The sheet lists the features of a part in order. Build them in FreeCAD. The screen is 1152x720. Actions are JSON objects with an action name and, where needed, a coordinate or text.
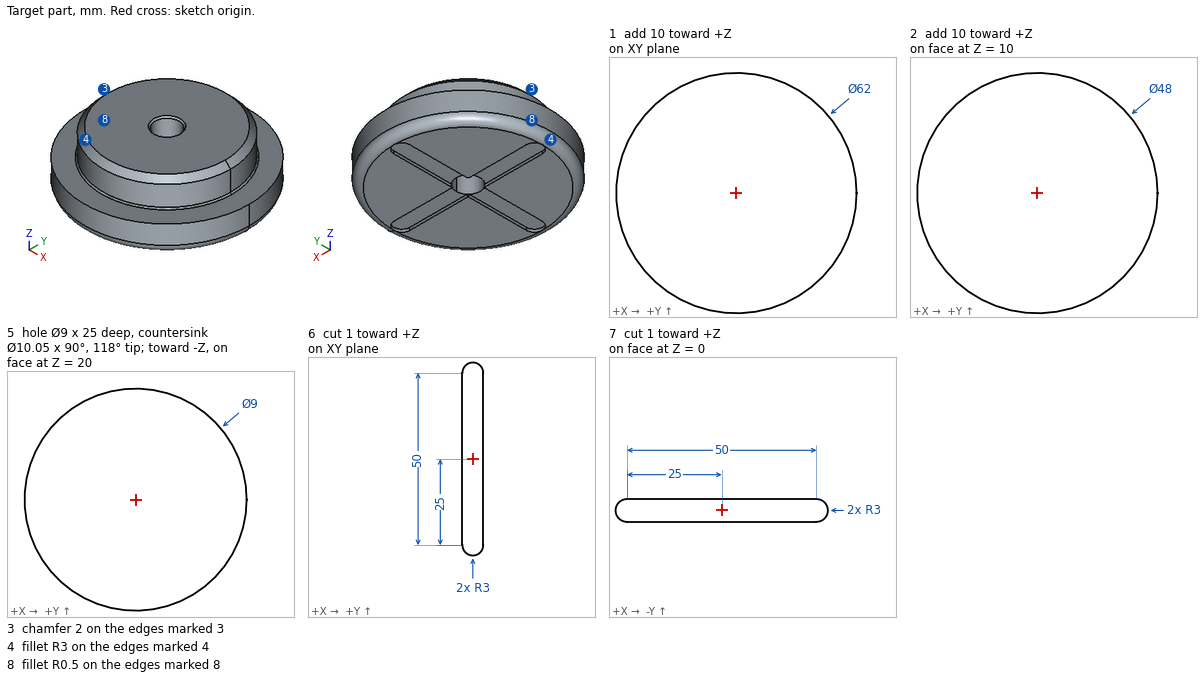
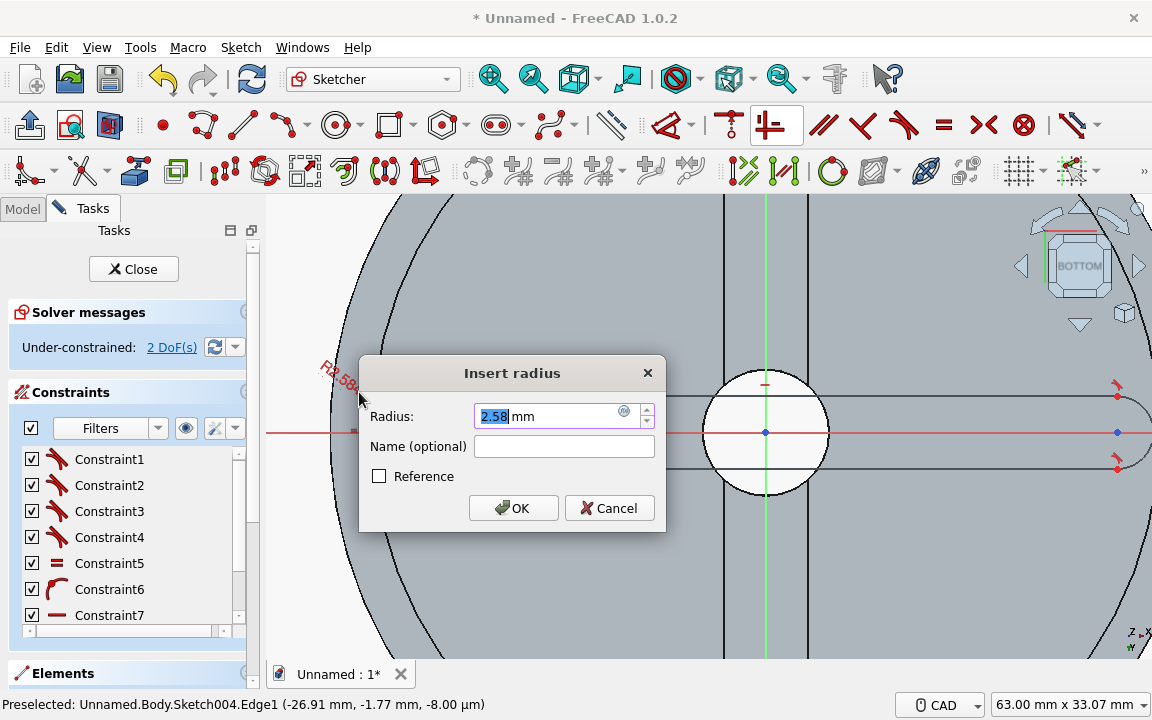
{"action": "type", "text": "3"}
{"action": "key", "text": "Return"}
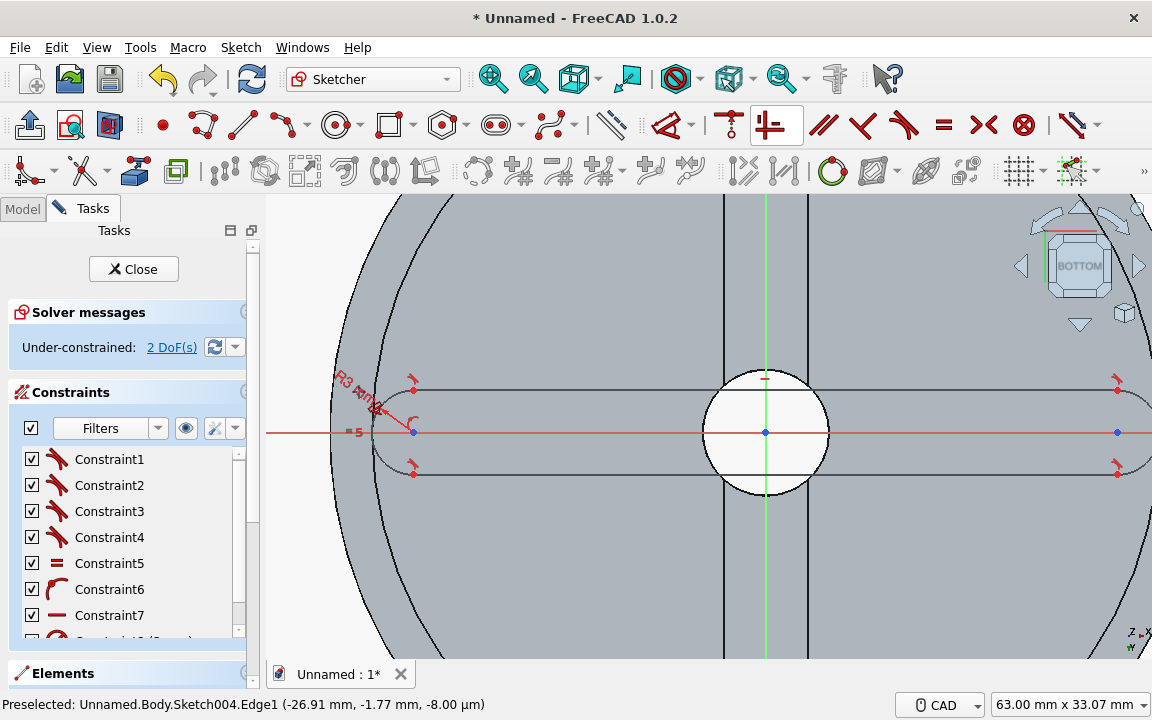
{"action": "left_click", "coordinate": [625, 390]}
{"action": "left_click", "coordinate": [700, 356]}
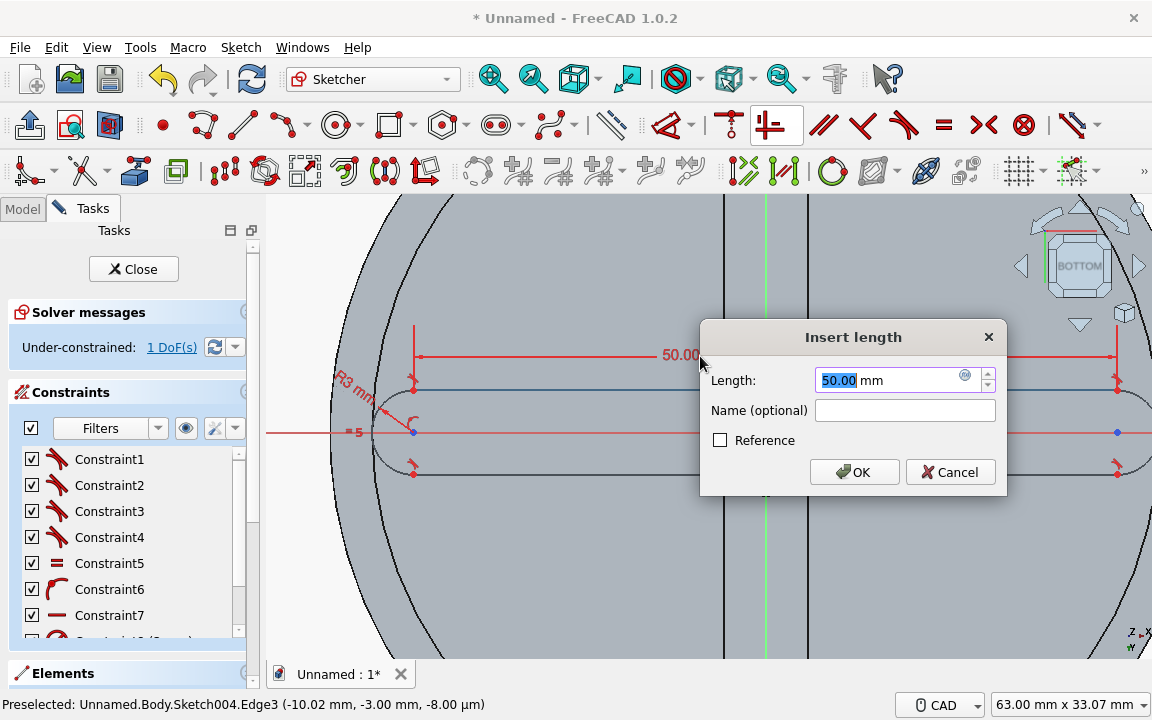
{"action": "type", "text": "50"}
{"action": "key", "text": "Return"}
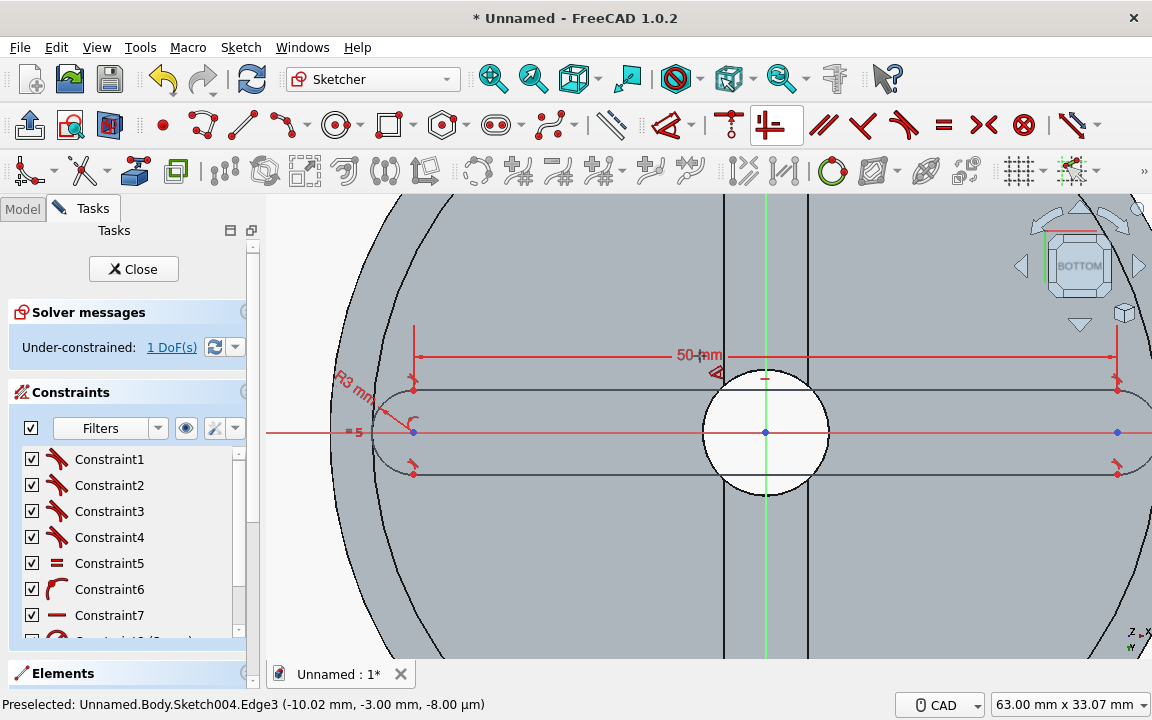
{"action": "left_click", "coordinate": [414, 390]}
{"action": "left_click", "coordinate": [590, 356]}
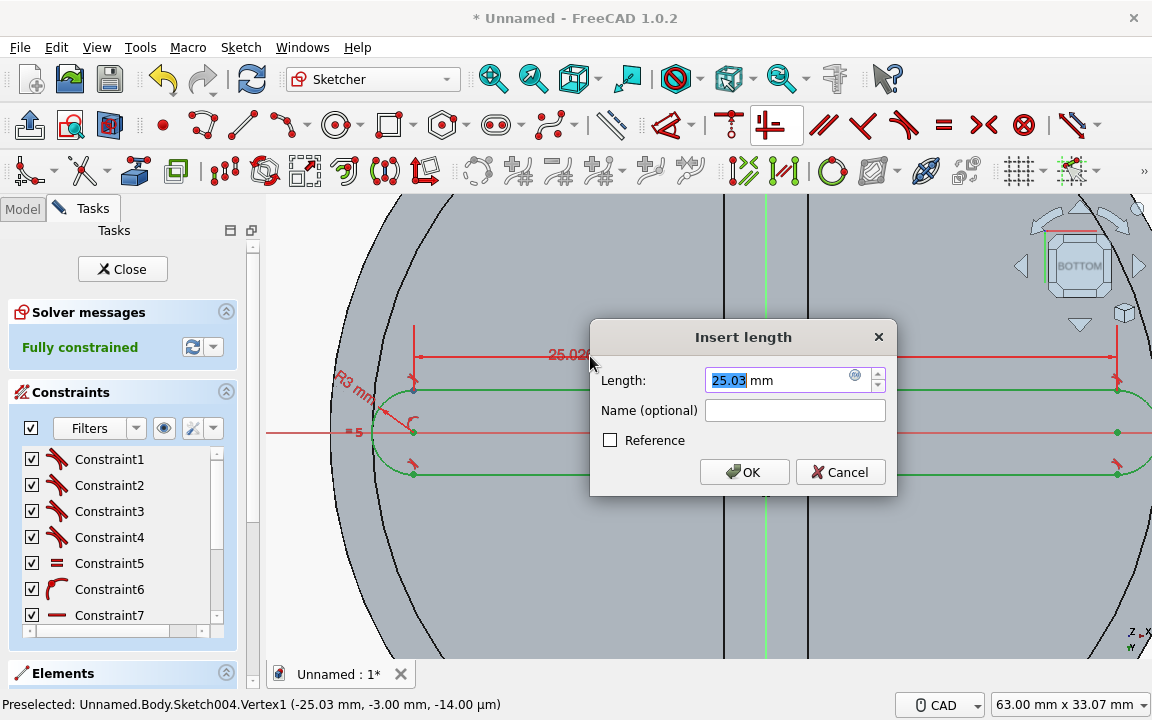
{"action": "type", "text": "25"}
{"action": "key", "text": "Return"}
{"action": "key", "text": "Escape"}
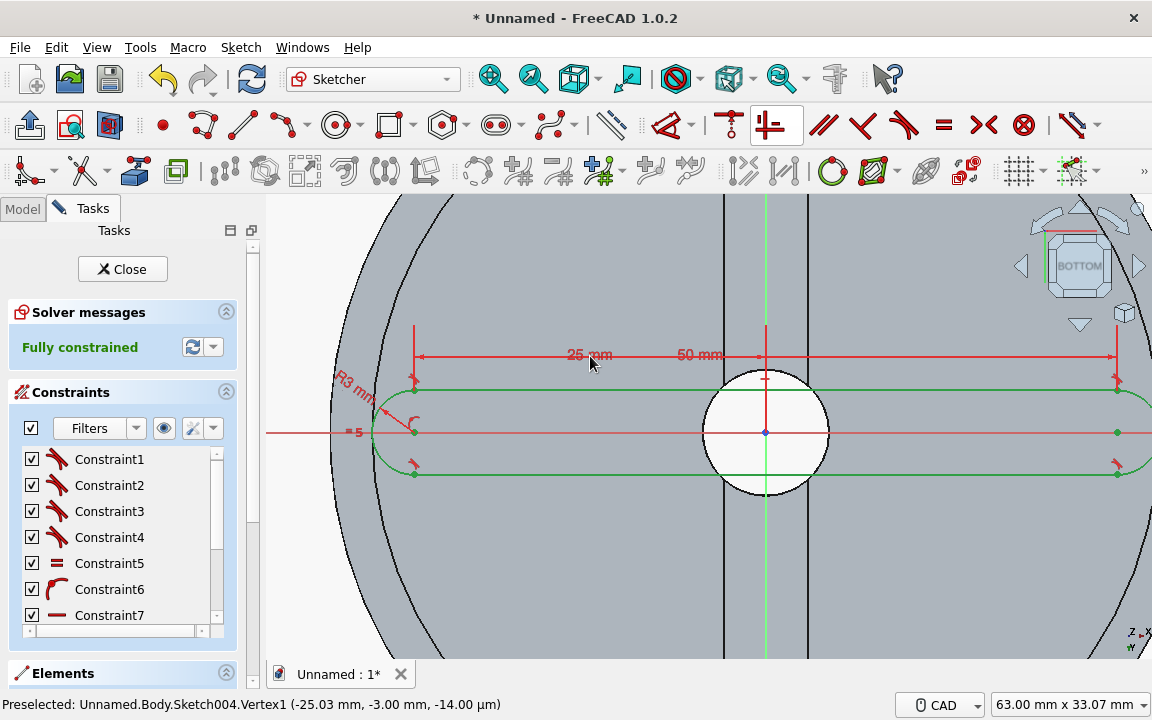
{"action": "left_click", "coordinate": [123, 269]}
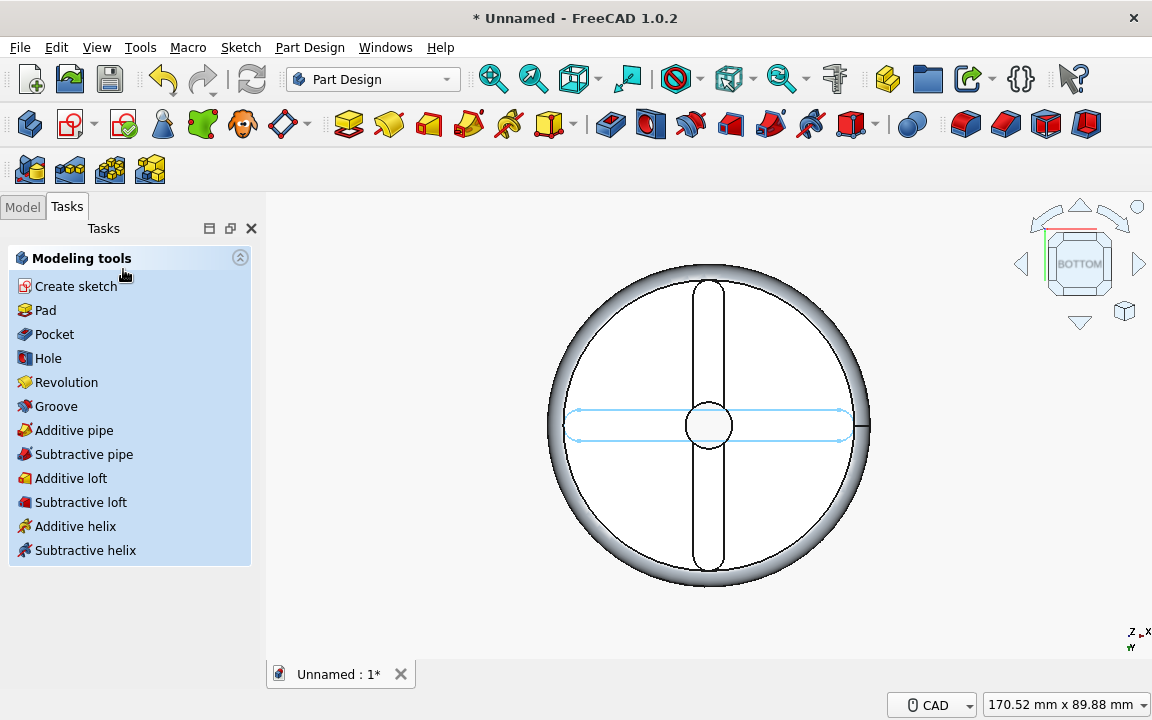
{"action": "left_click", "coordinate": [612, 124]}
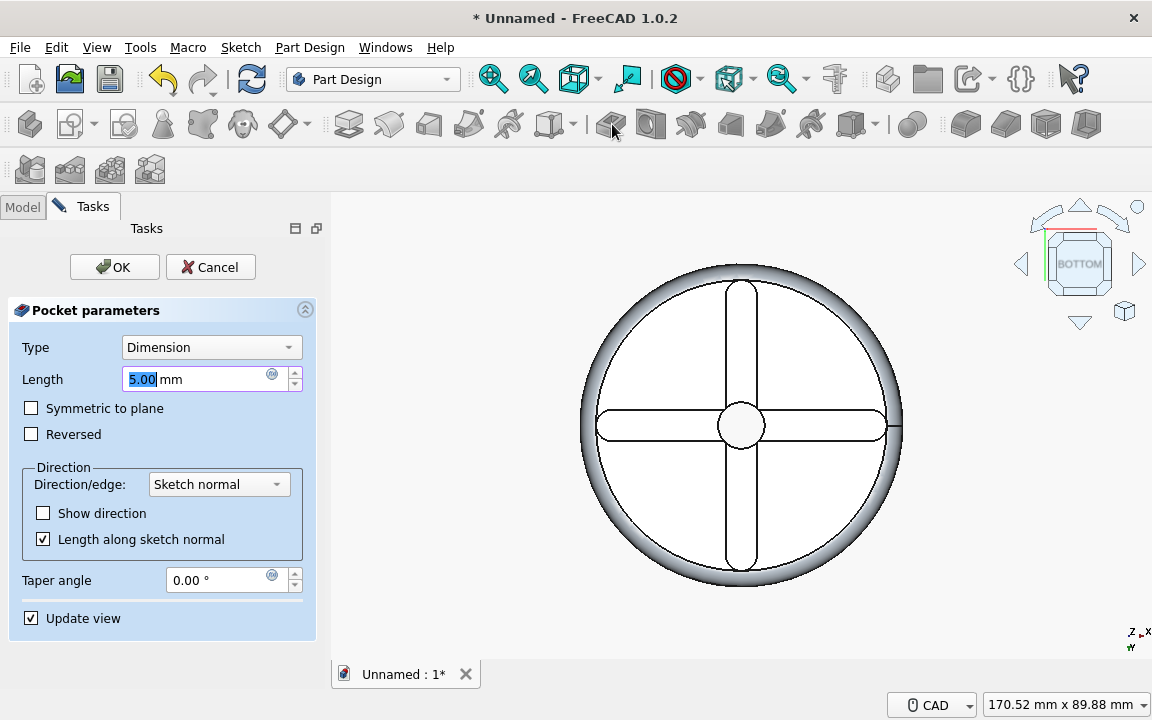
{"action": "type", "text": "1"}
{"action": "key", "text": "Tab"}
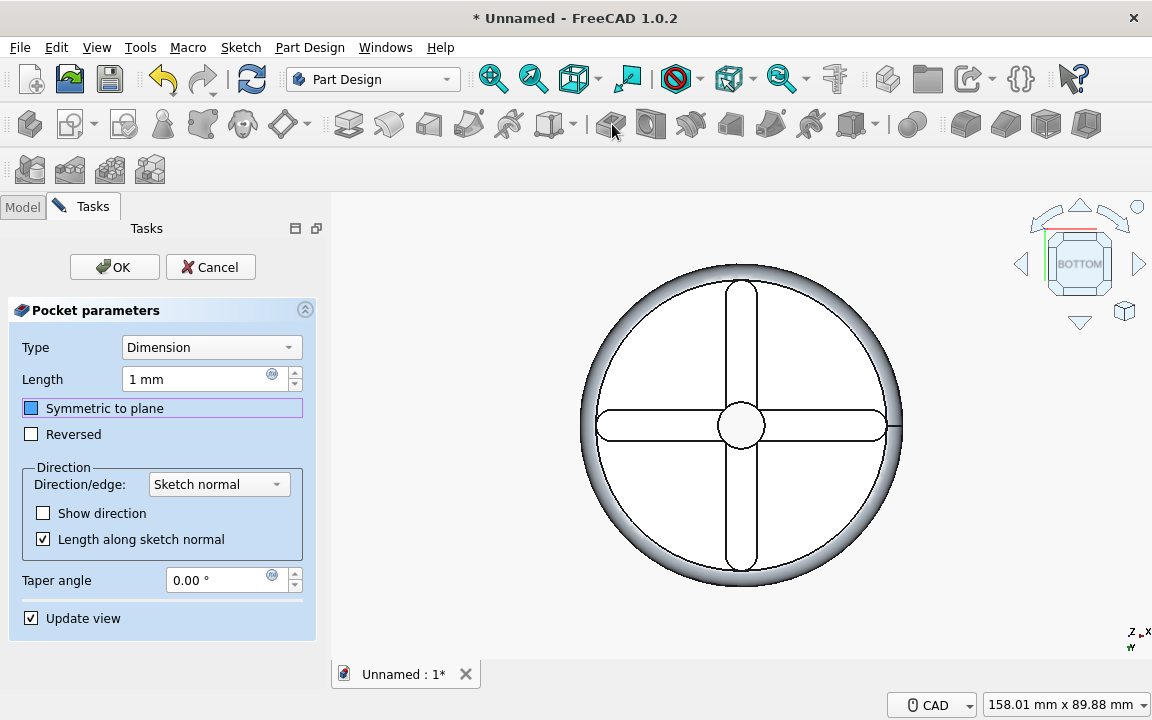
{"action": "left_click", "coordinate": [115, 267]}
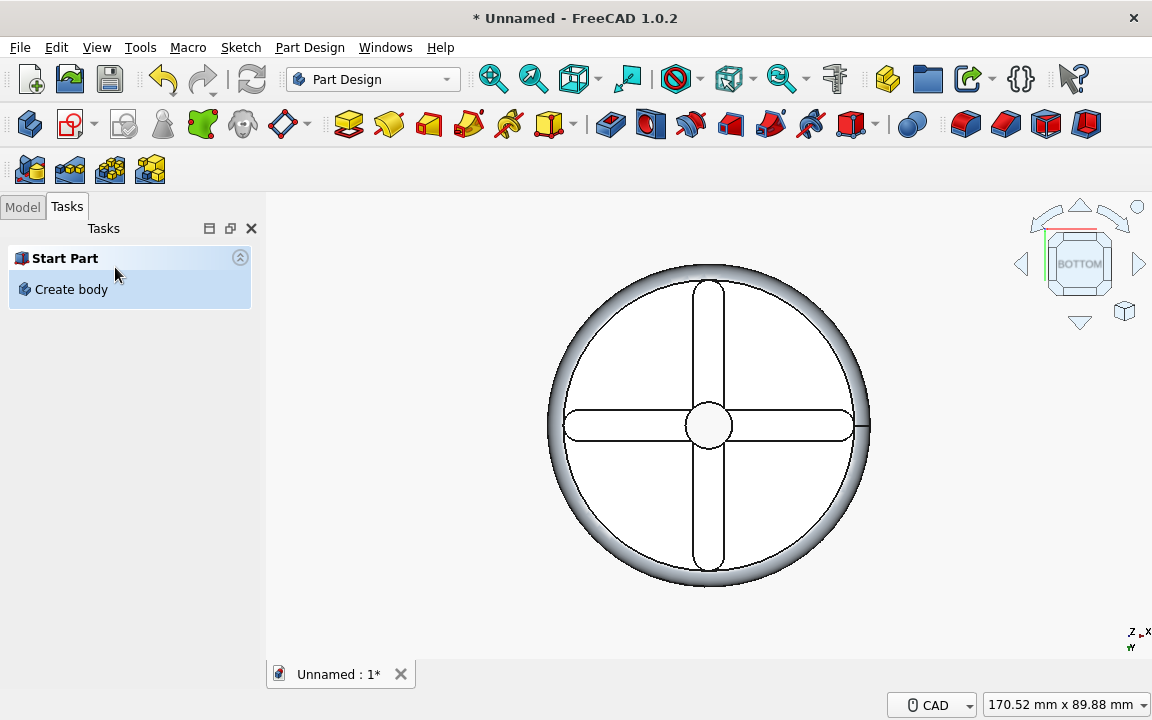
{"action": "key", "text": "0"}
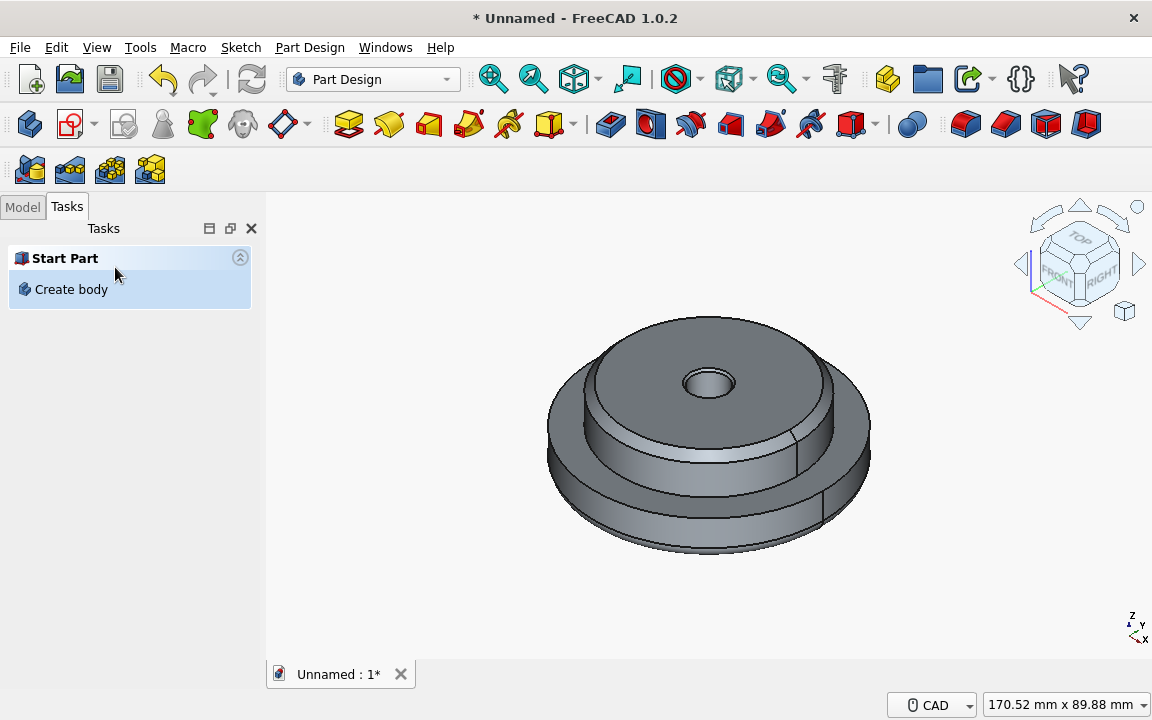
{"action": "key", "text": "2"}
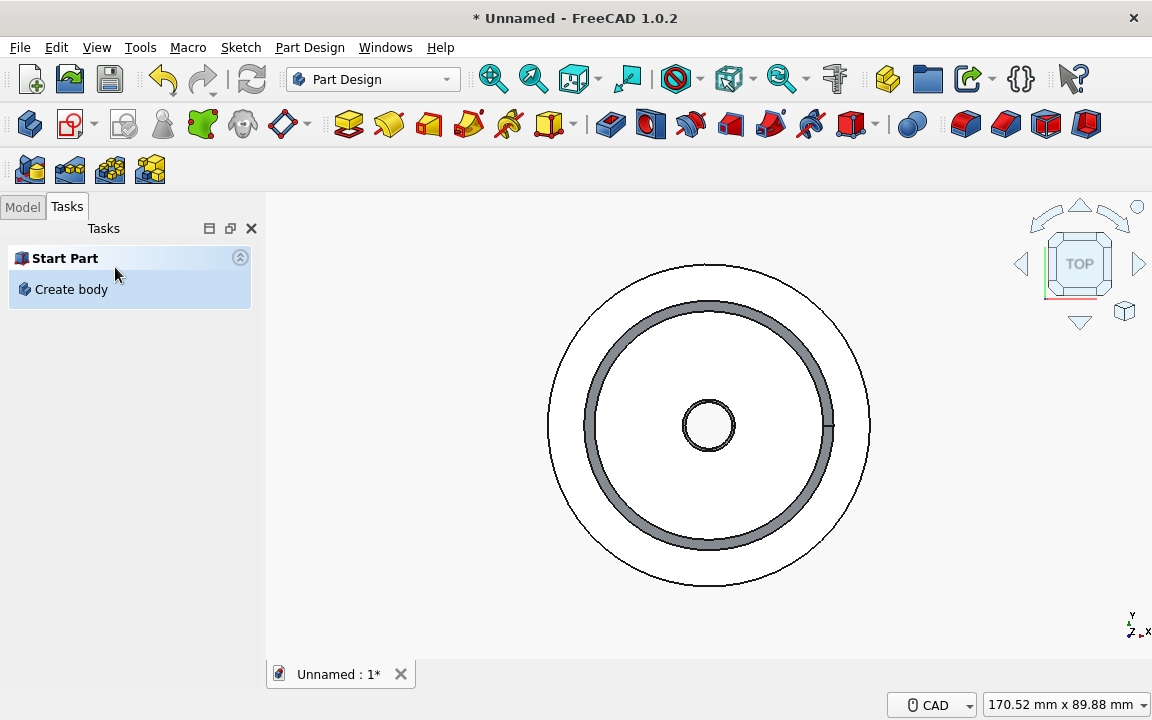
{"action": "key", "text": "1"}